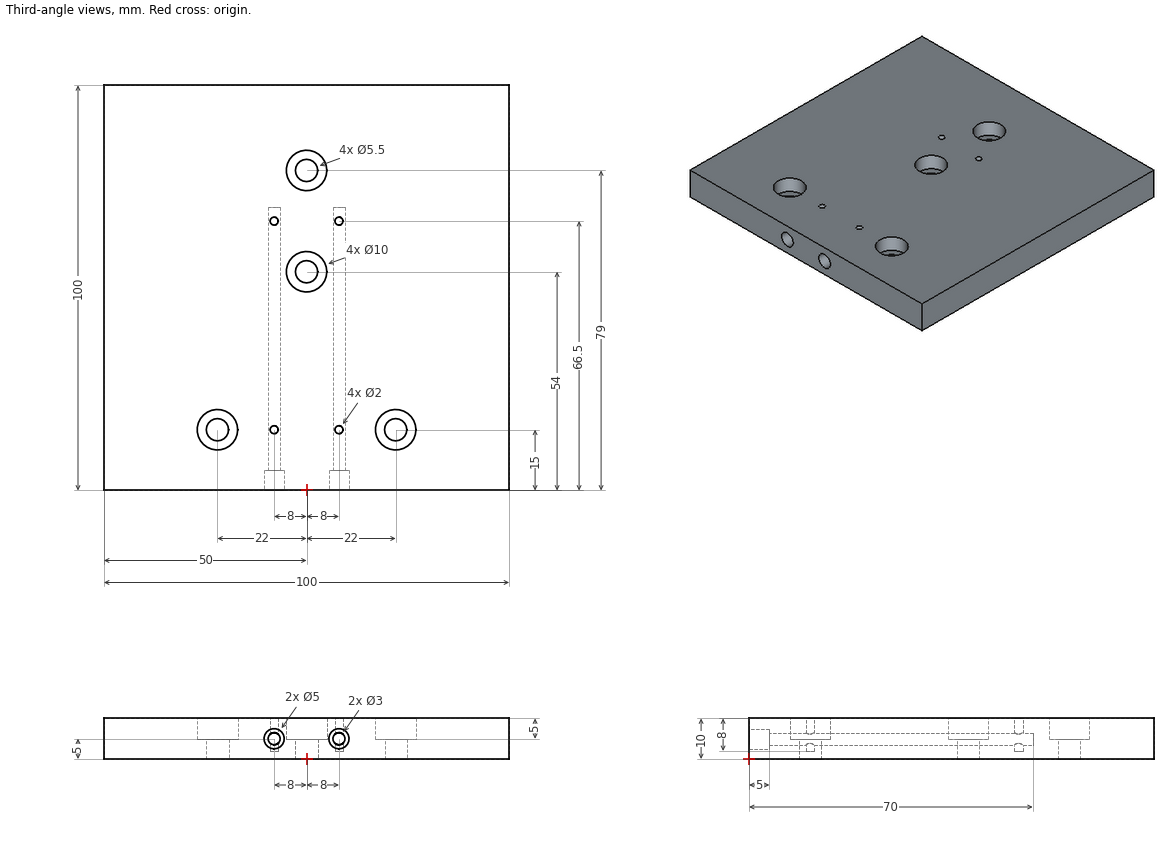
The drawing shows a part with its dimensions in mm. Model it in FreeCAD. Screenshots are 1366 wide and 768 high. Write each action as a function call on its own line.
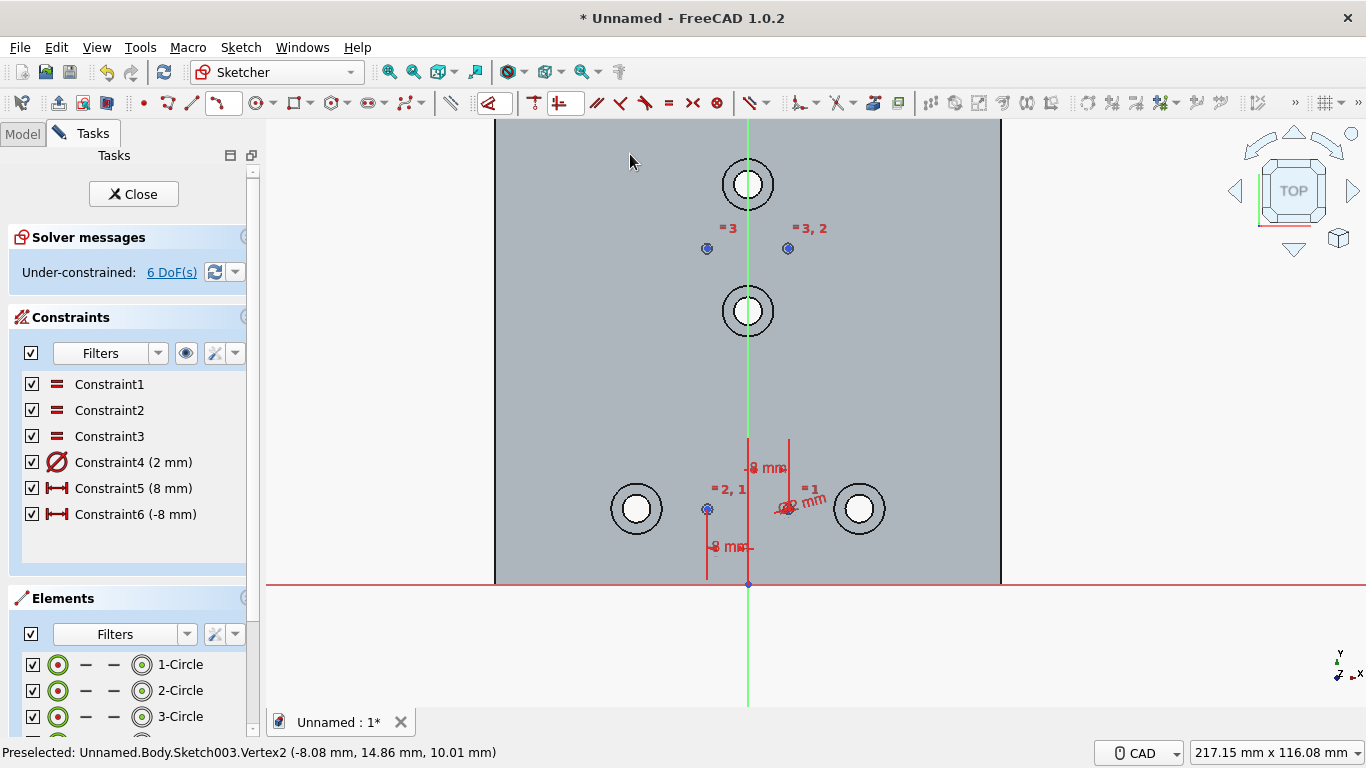
click(788, 248)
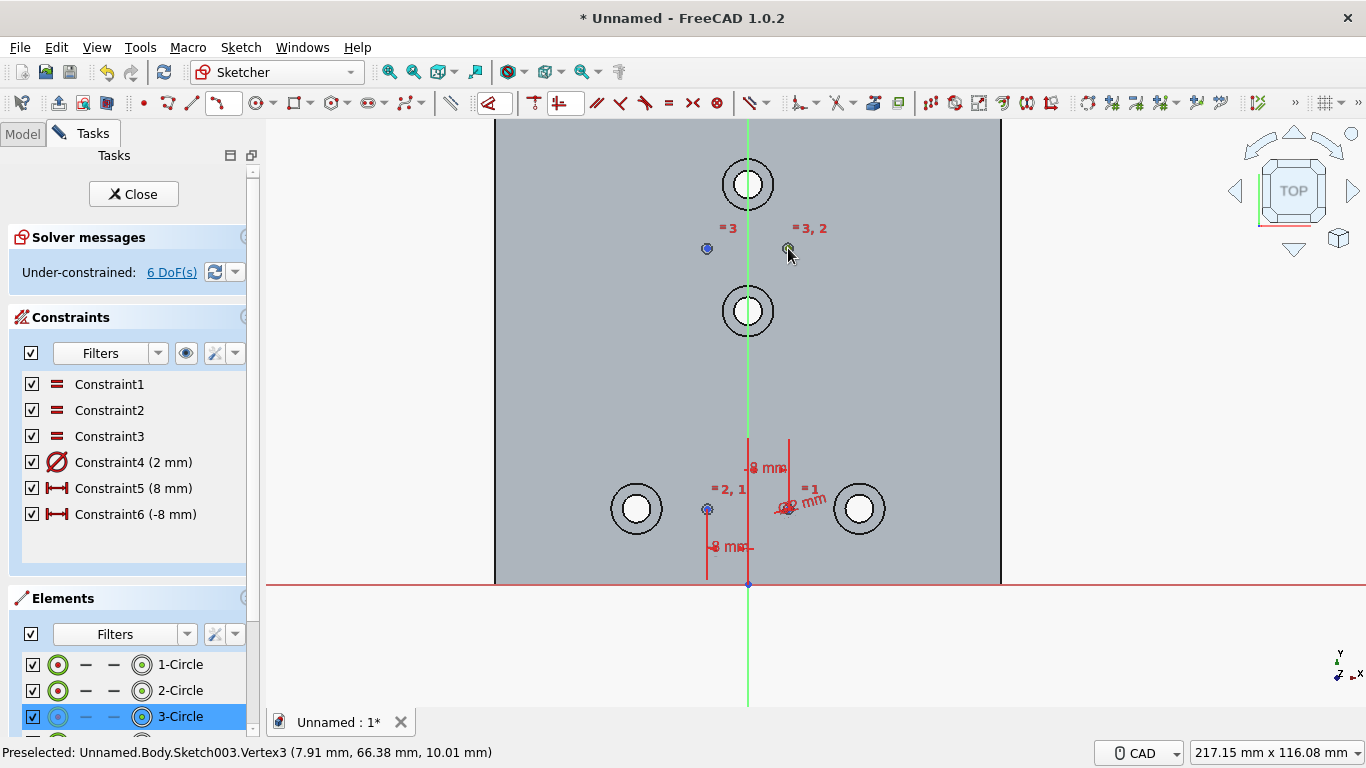
click(506, 104)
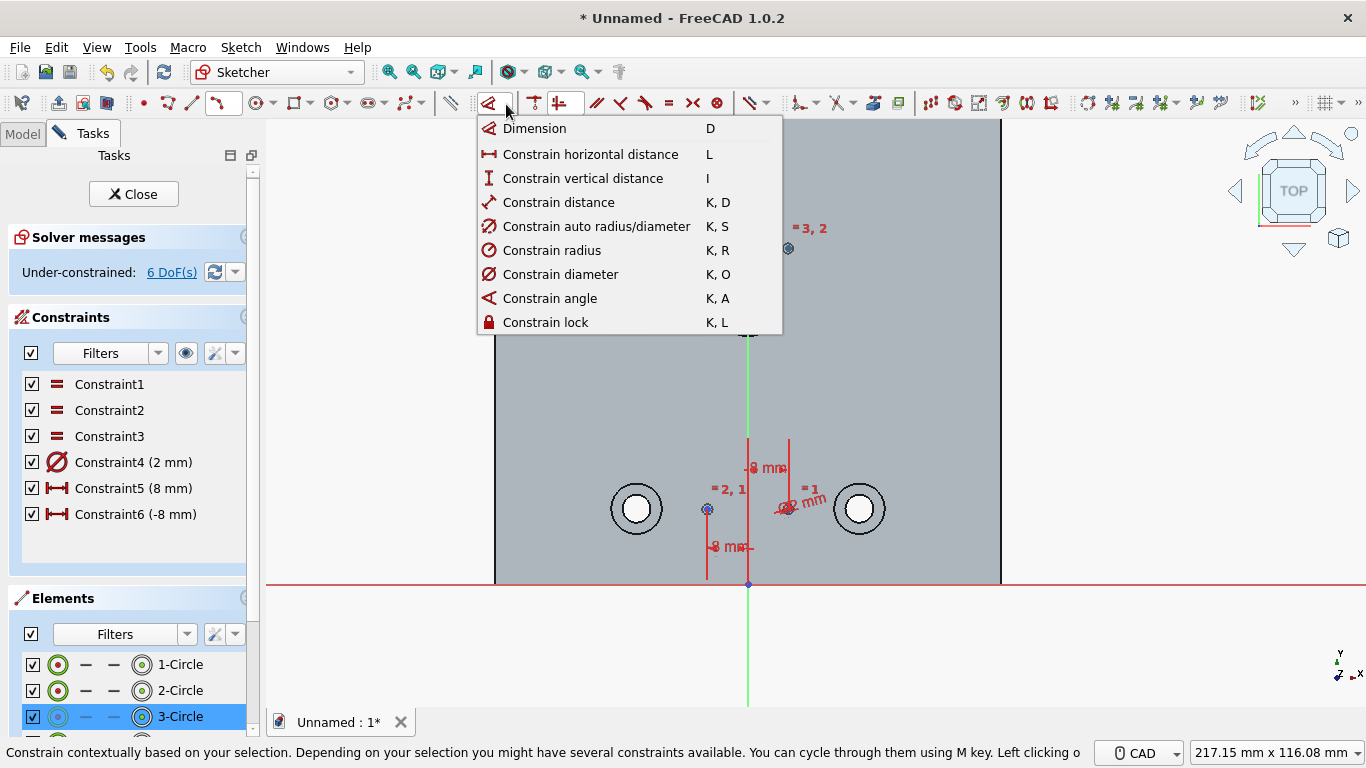
click(630, 154)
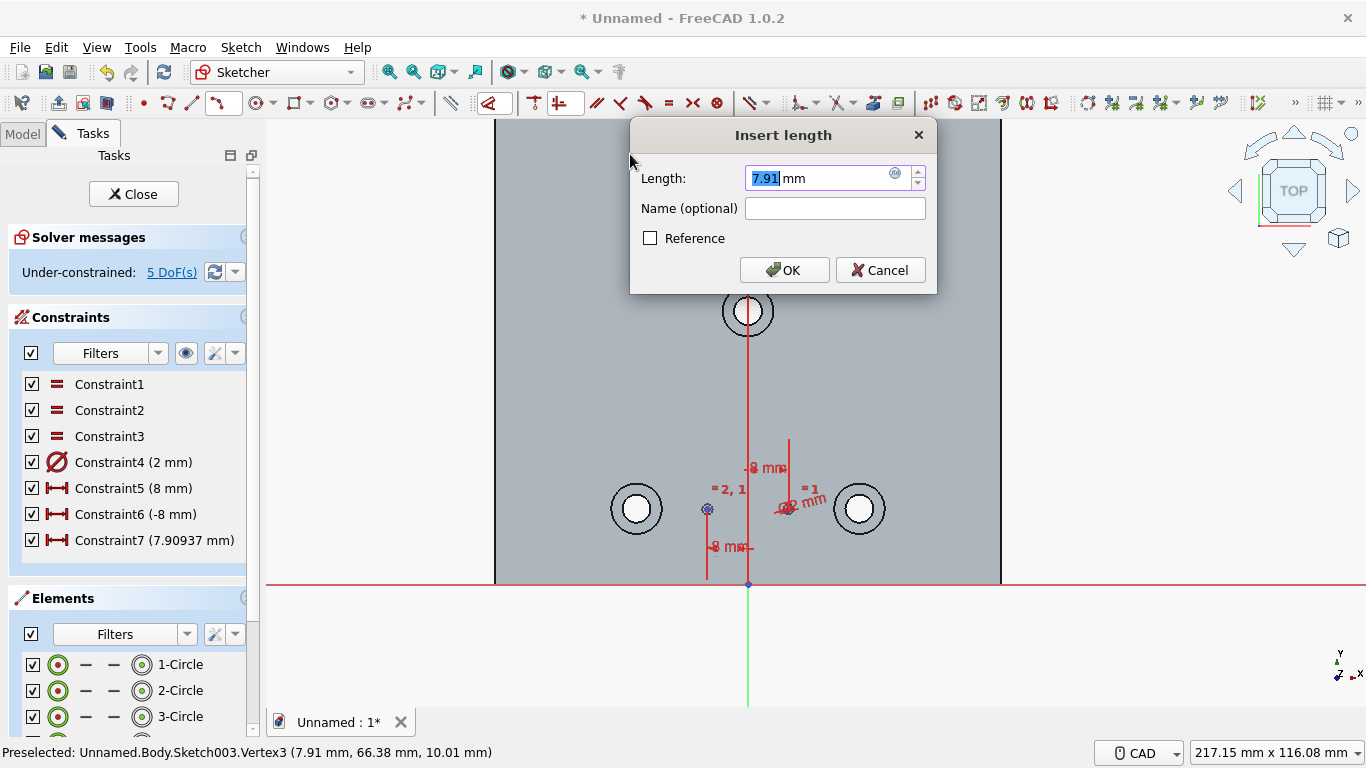
text(8)
key(Return)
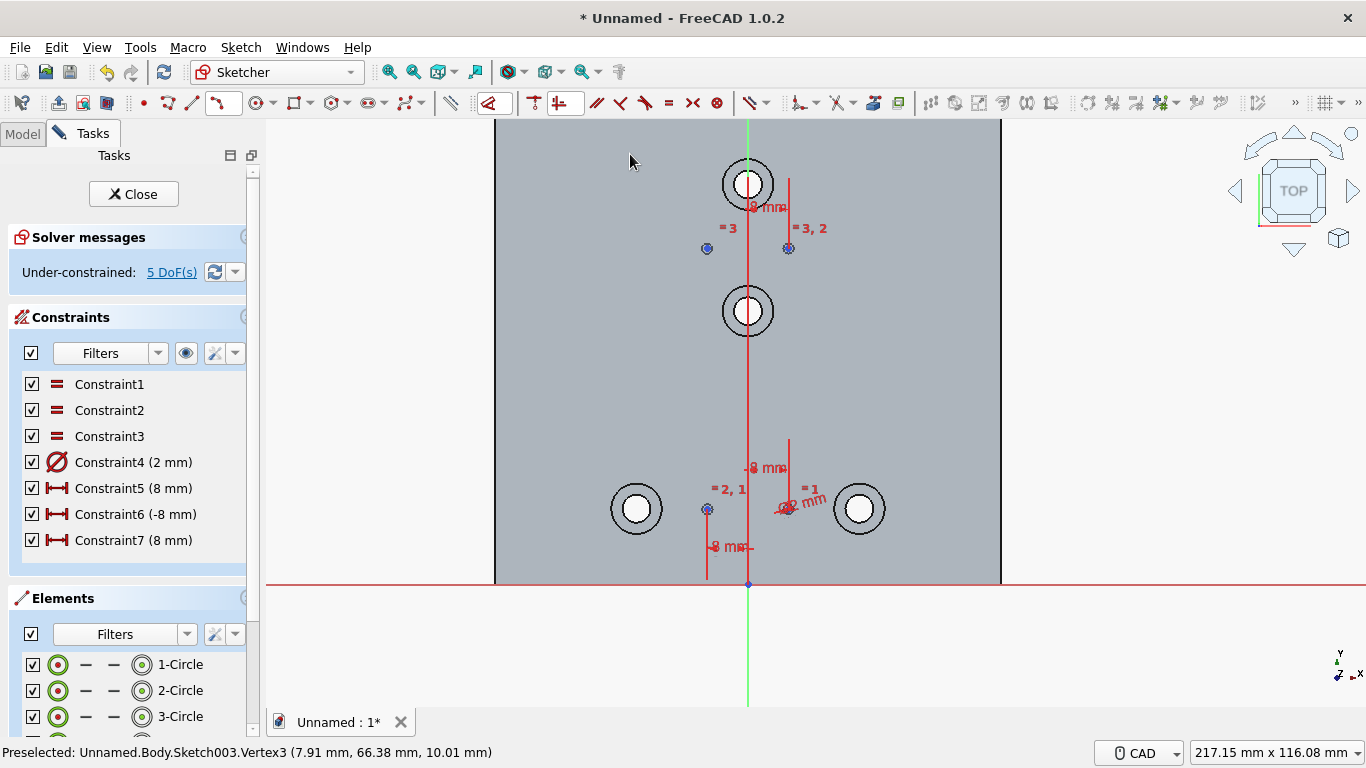
click(707, 249)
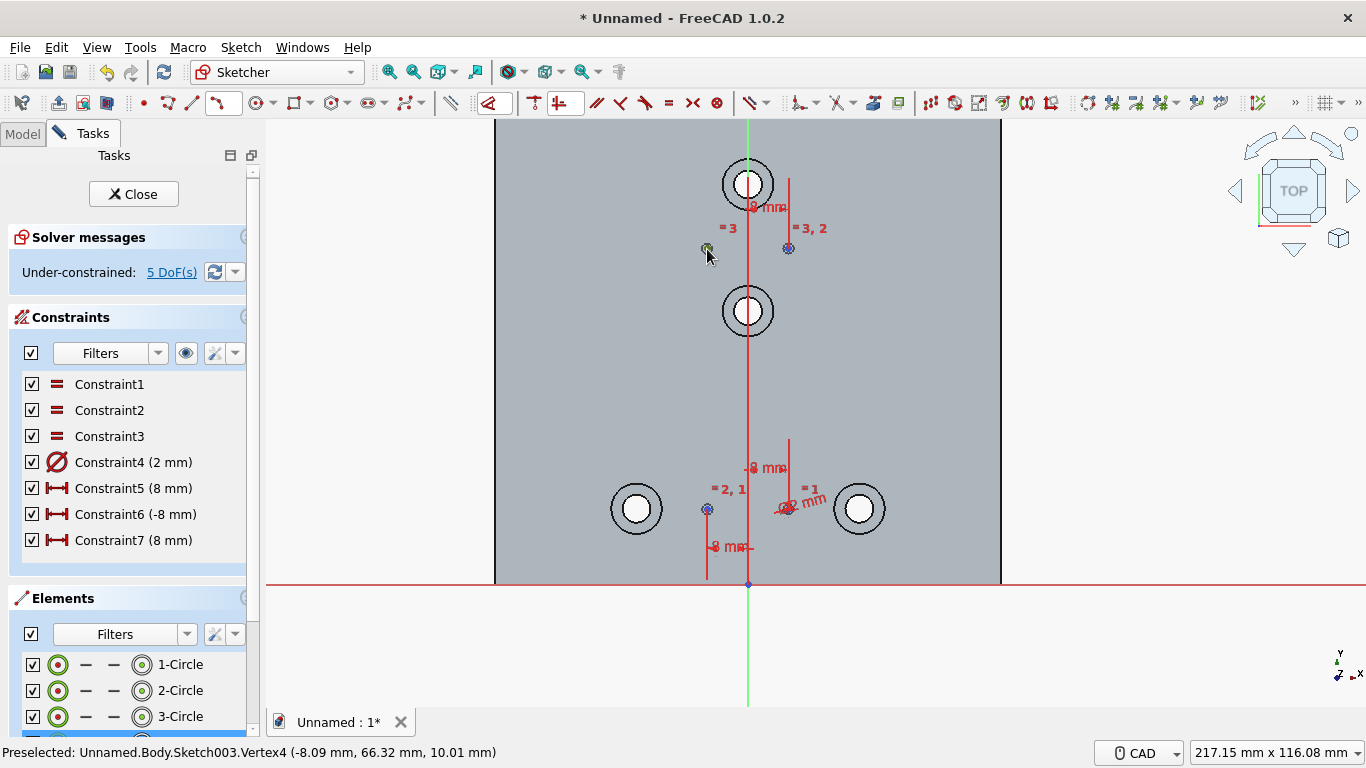
click(506, 104)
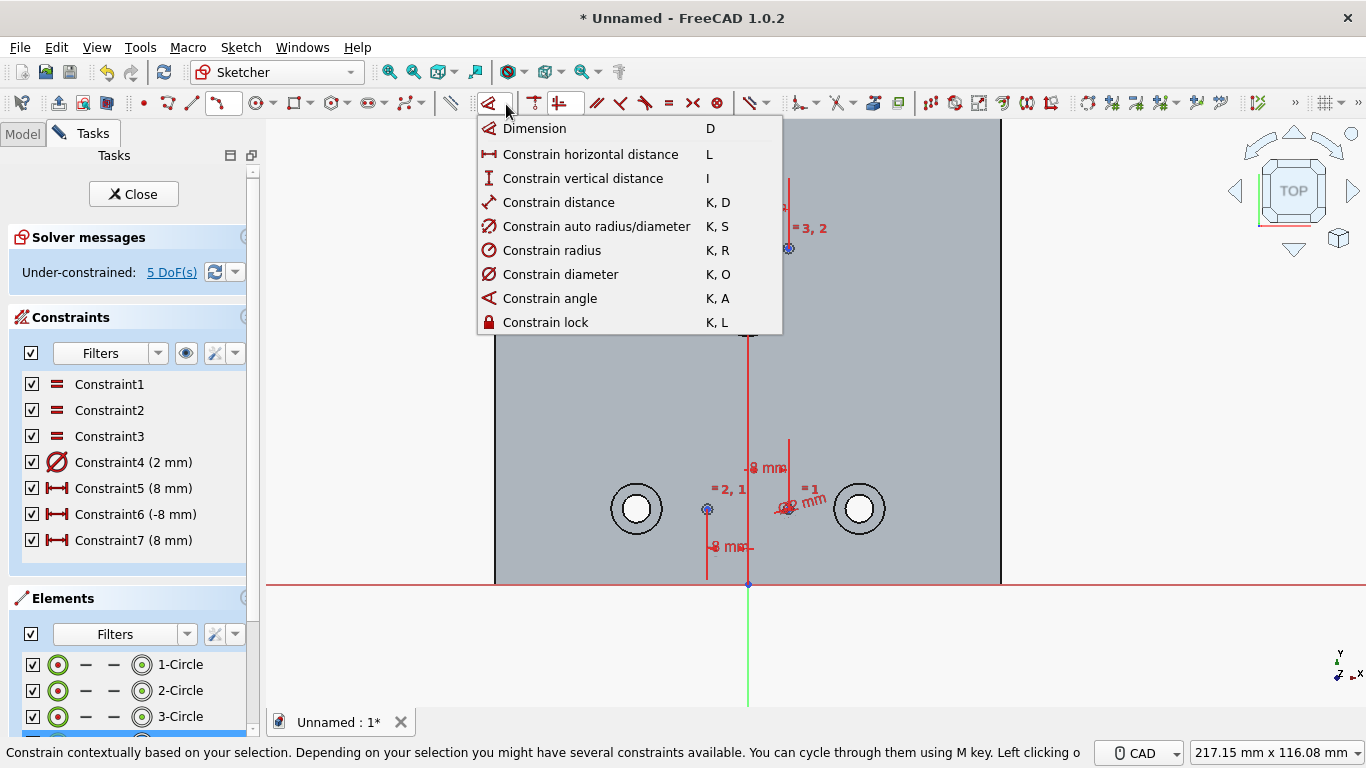
click(630, 154)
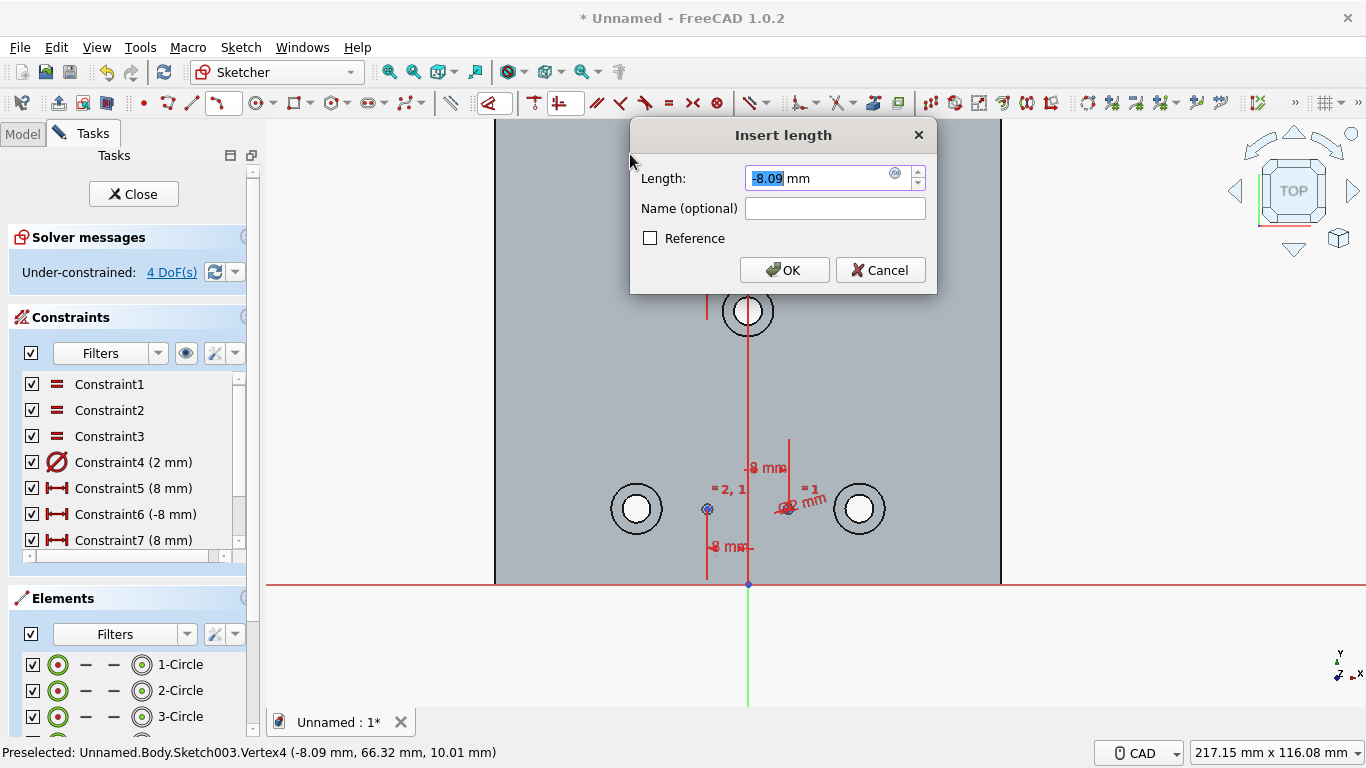
text(-8)
key(Return)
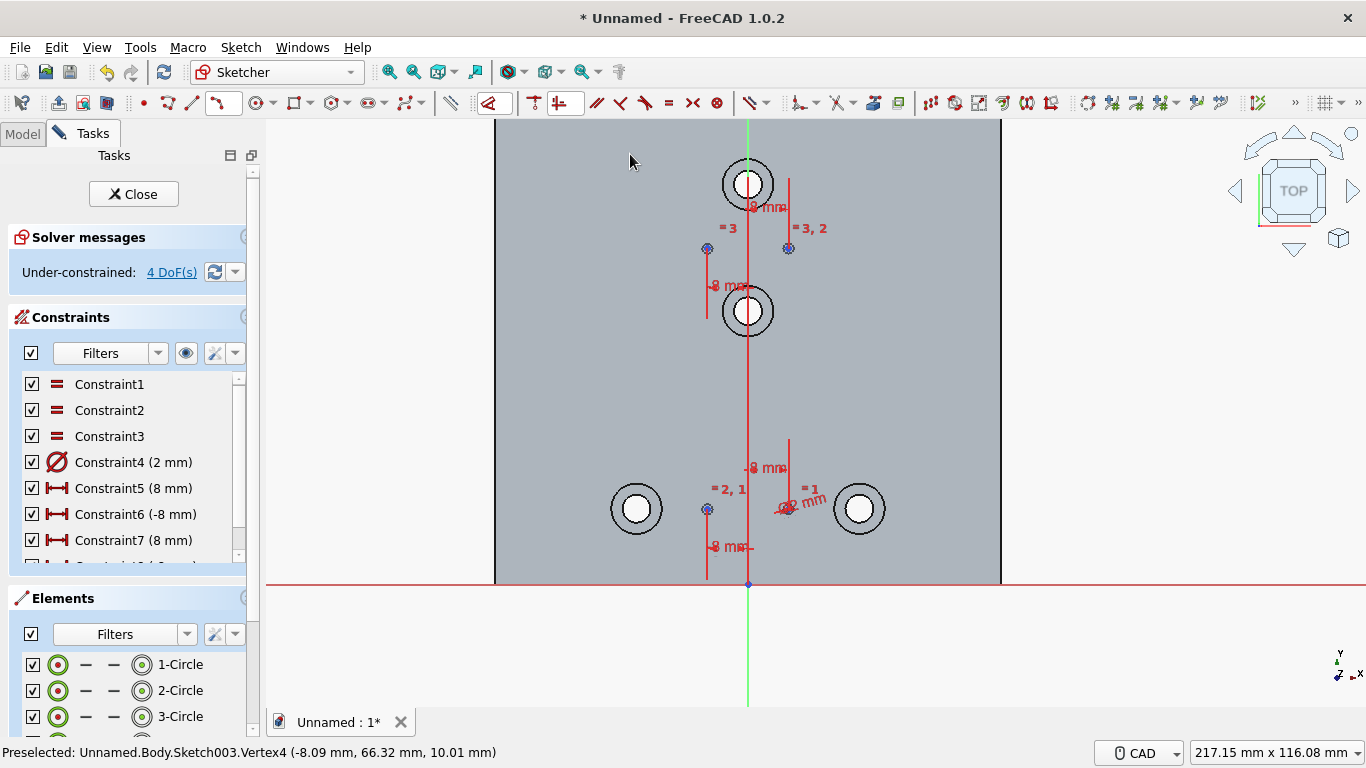
click(789, 509)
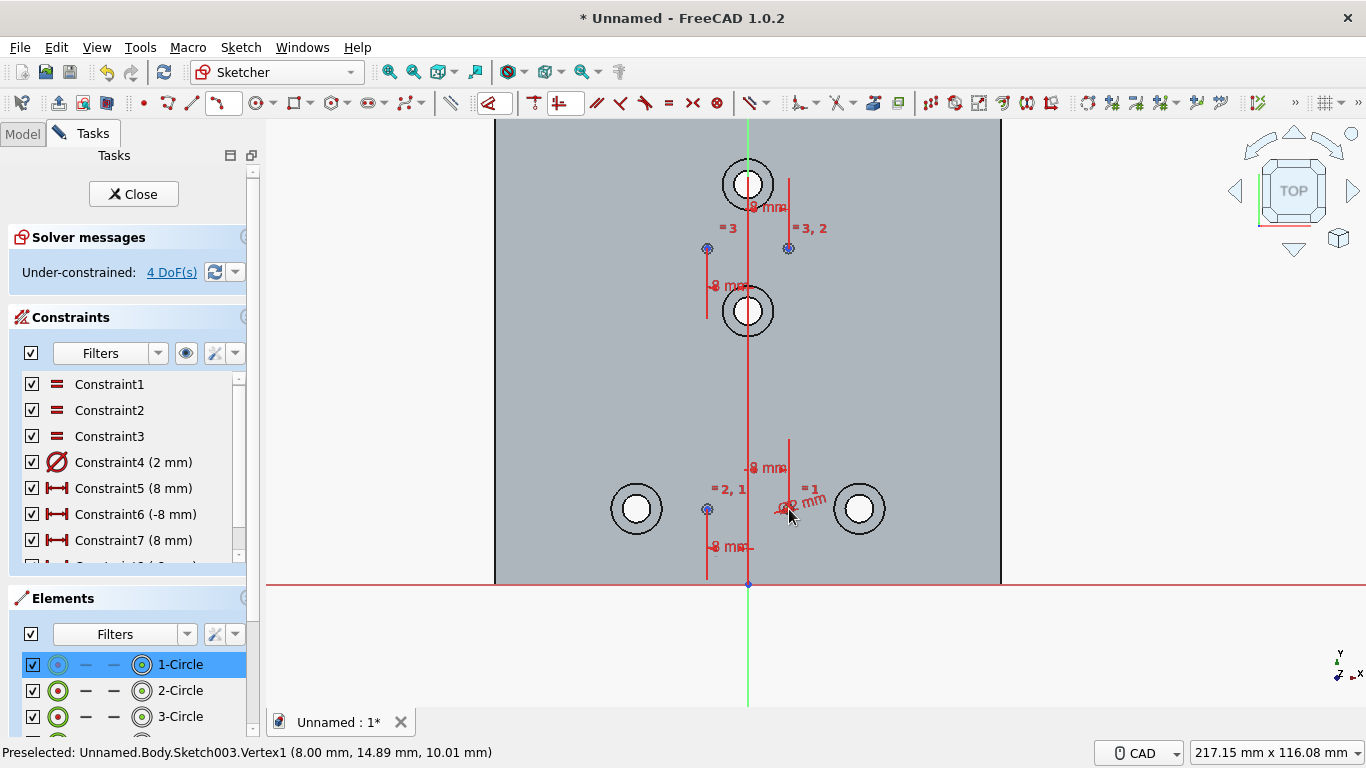
click(506, 104)